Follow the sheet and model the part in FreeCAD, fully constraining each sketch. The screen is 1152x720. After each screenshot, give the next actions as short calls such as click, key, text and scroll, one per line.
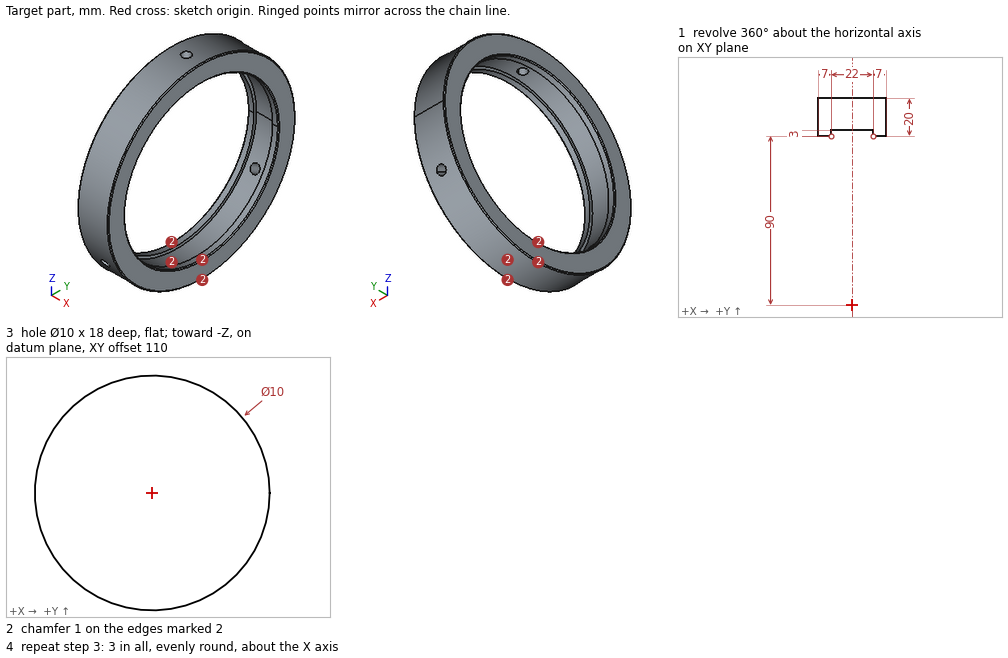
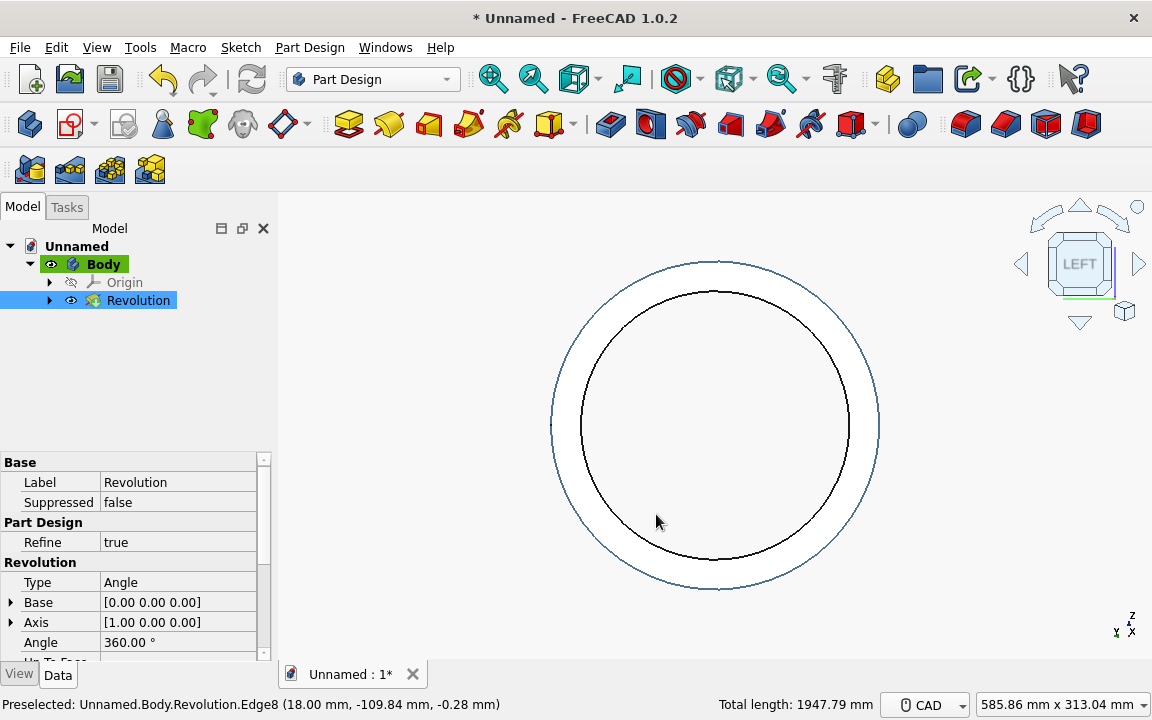
click(849, 424, ctrl)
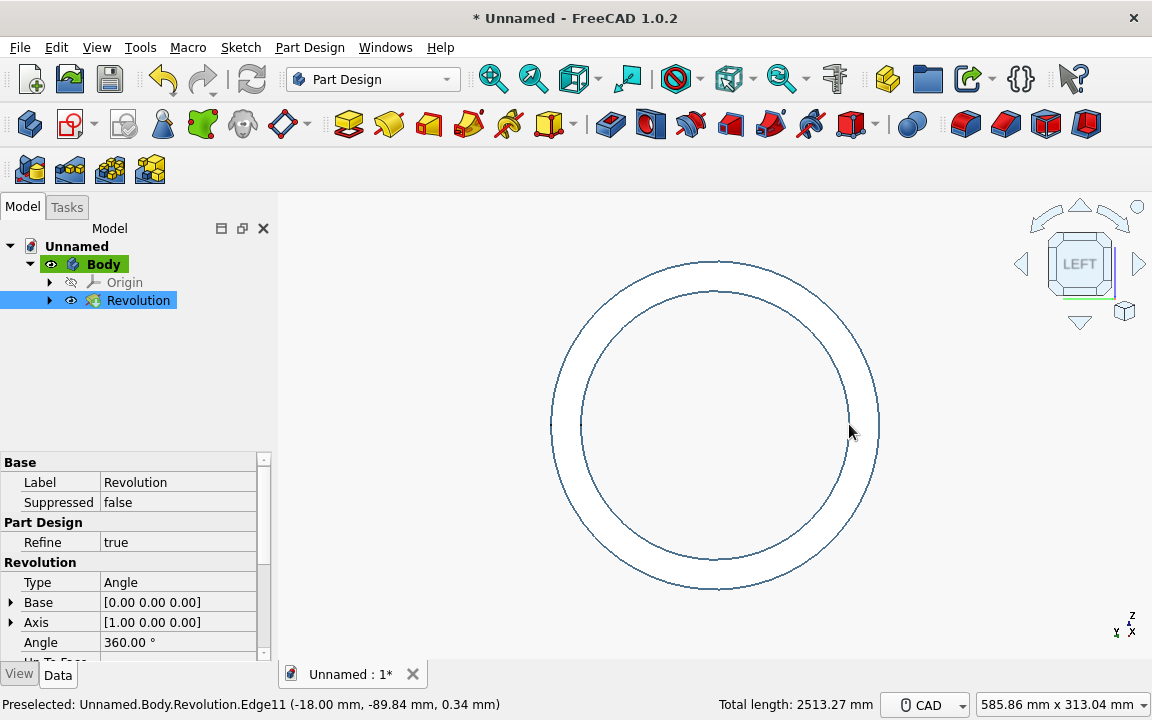
click(1006, 124)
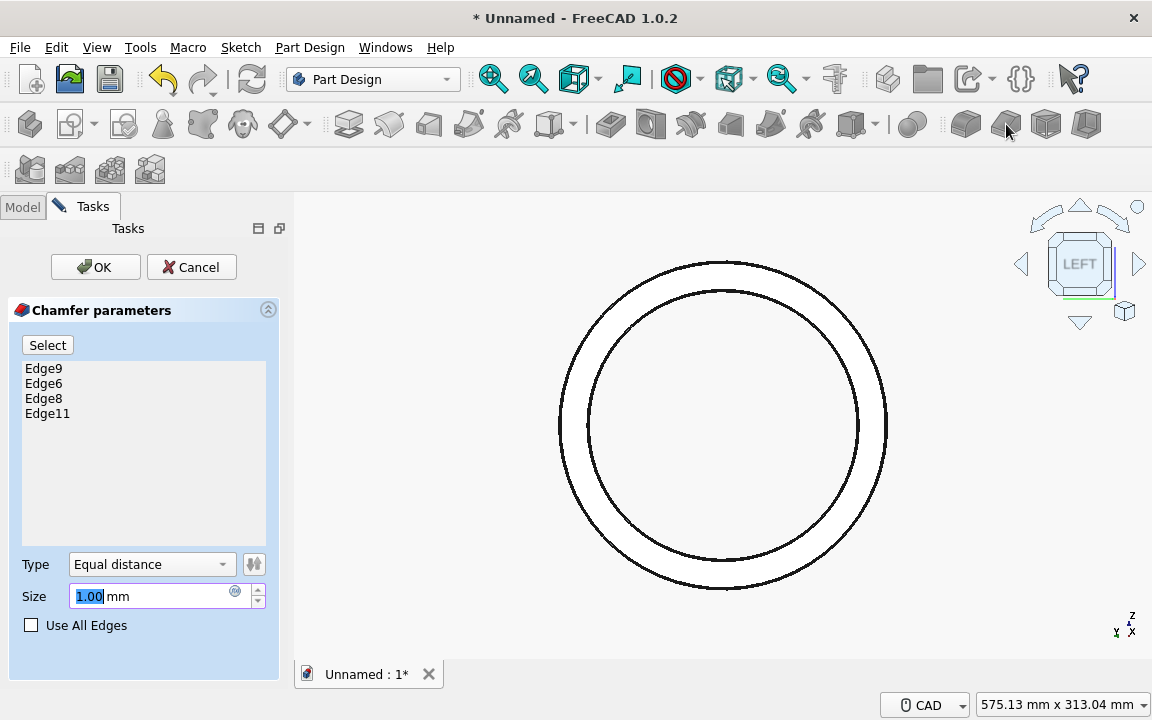
text(1)
key(Tab)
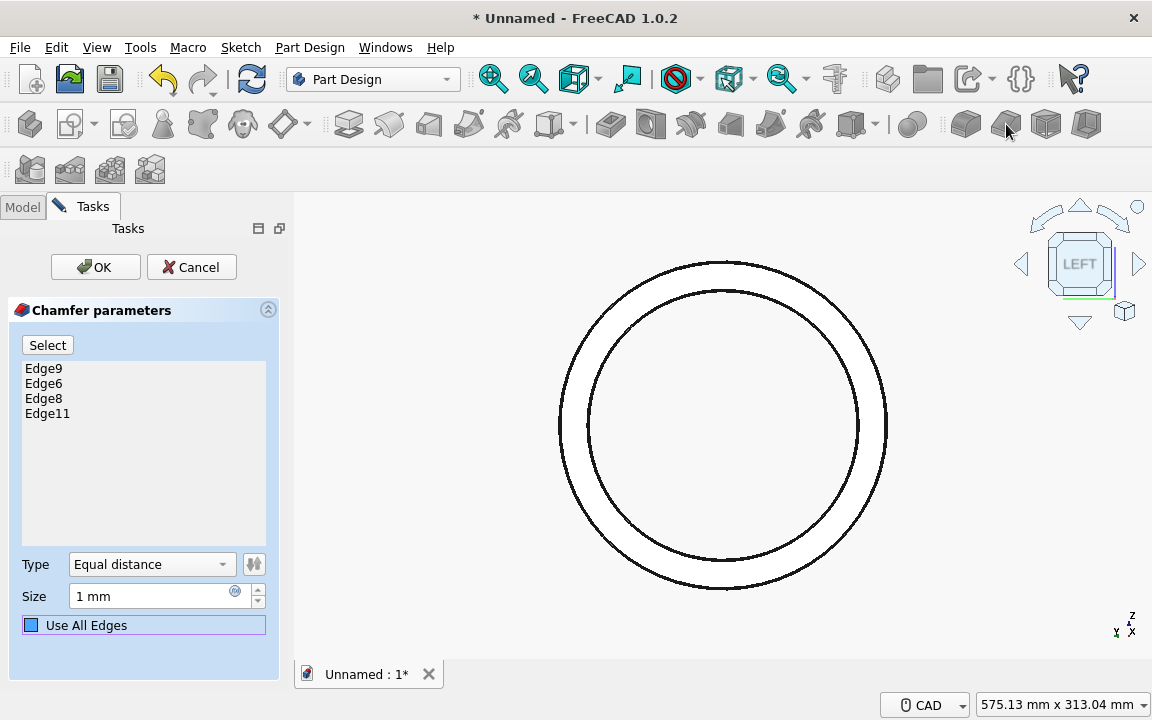
click(96, 267)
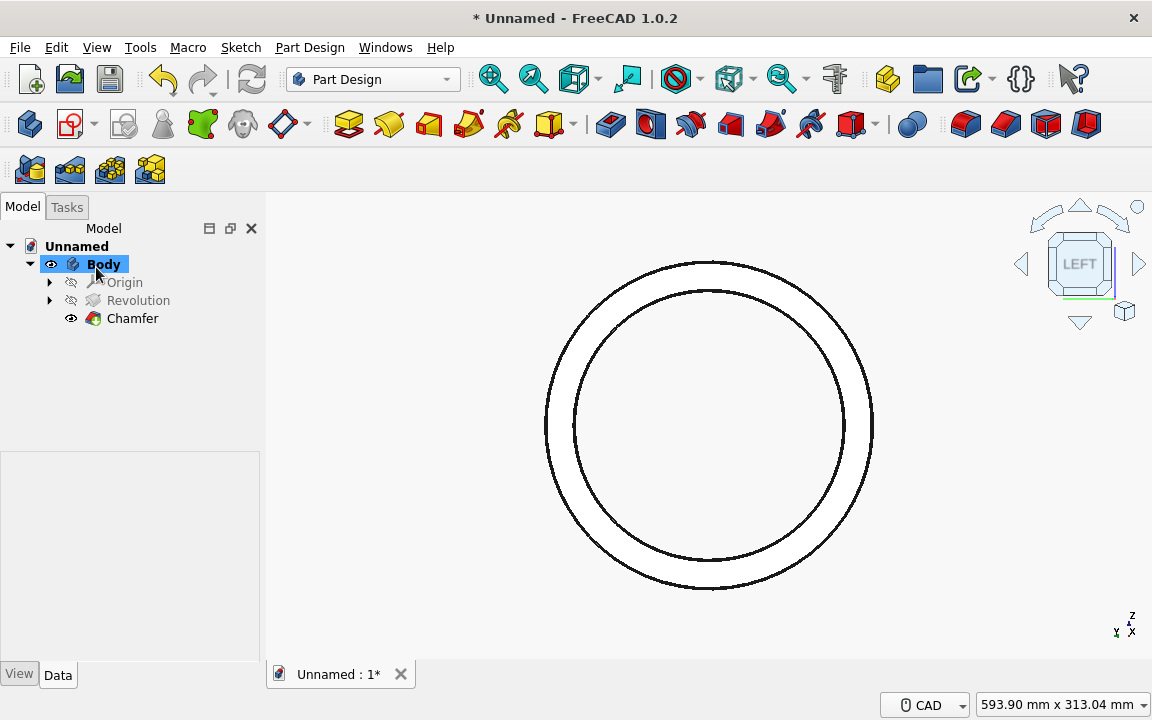
click(50, 282)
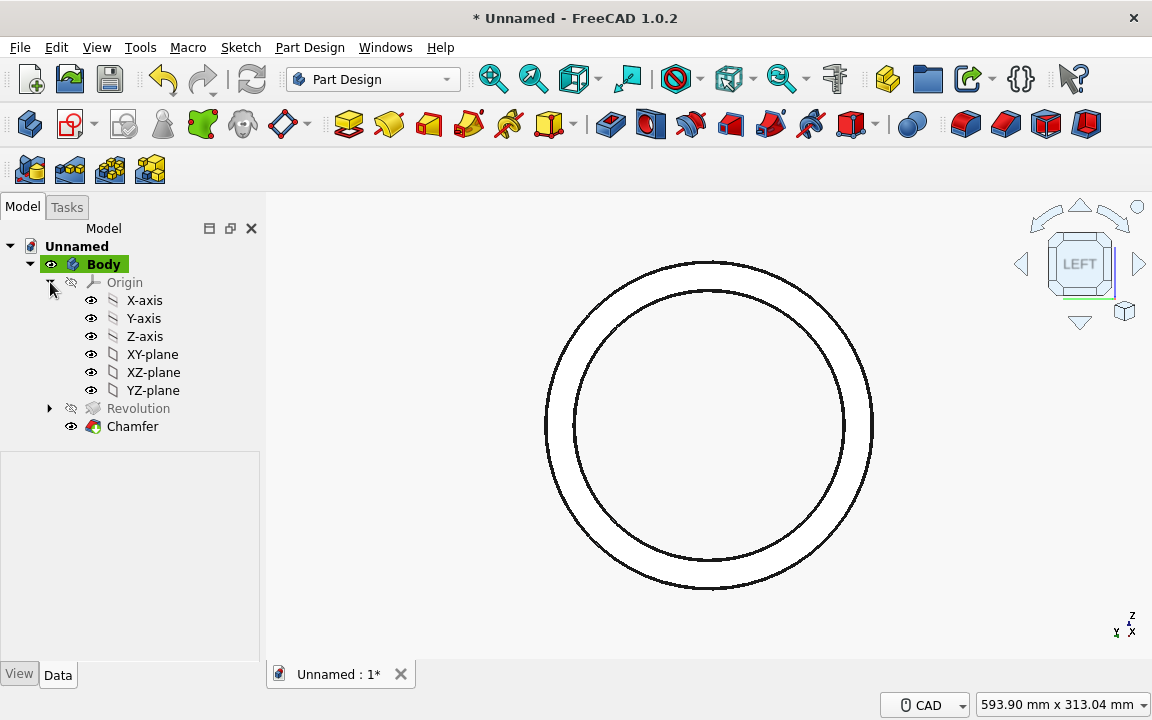
click(136, 354)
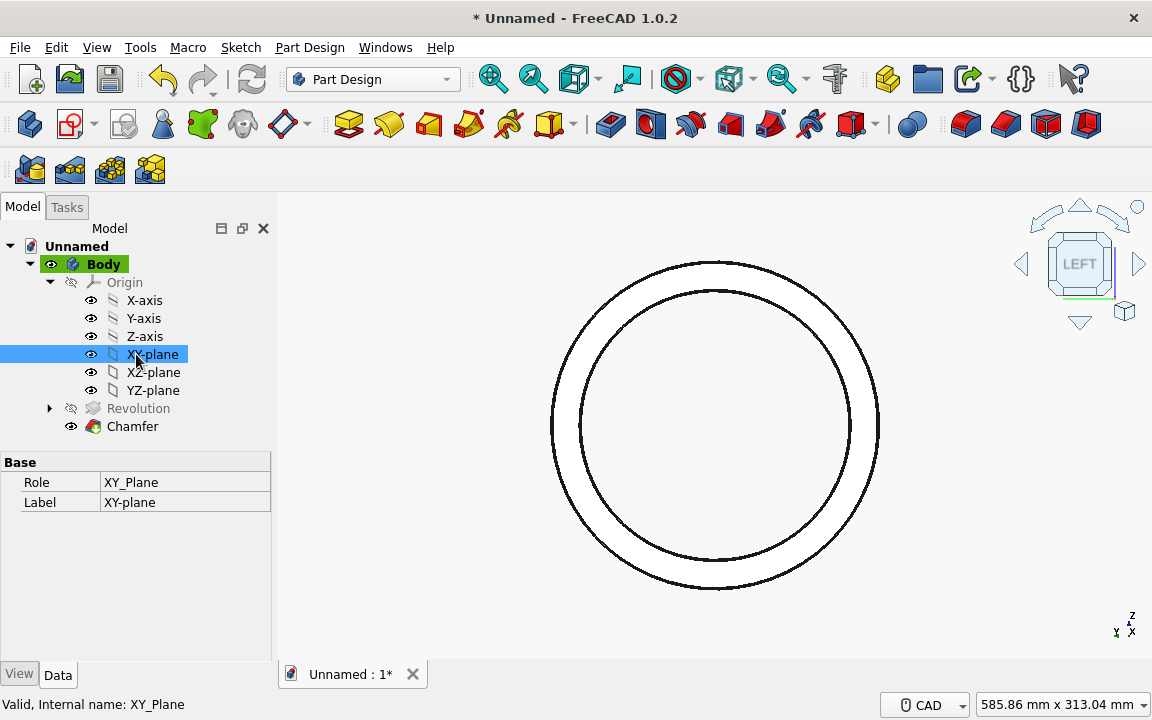
click(284, 124)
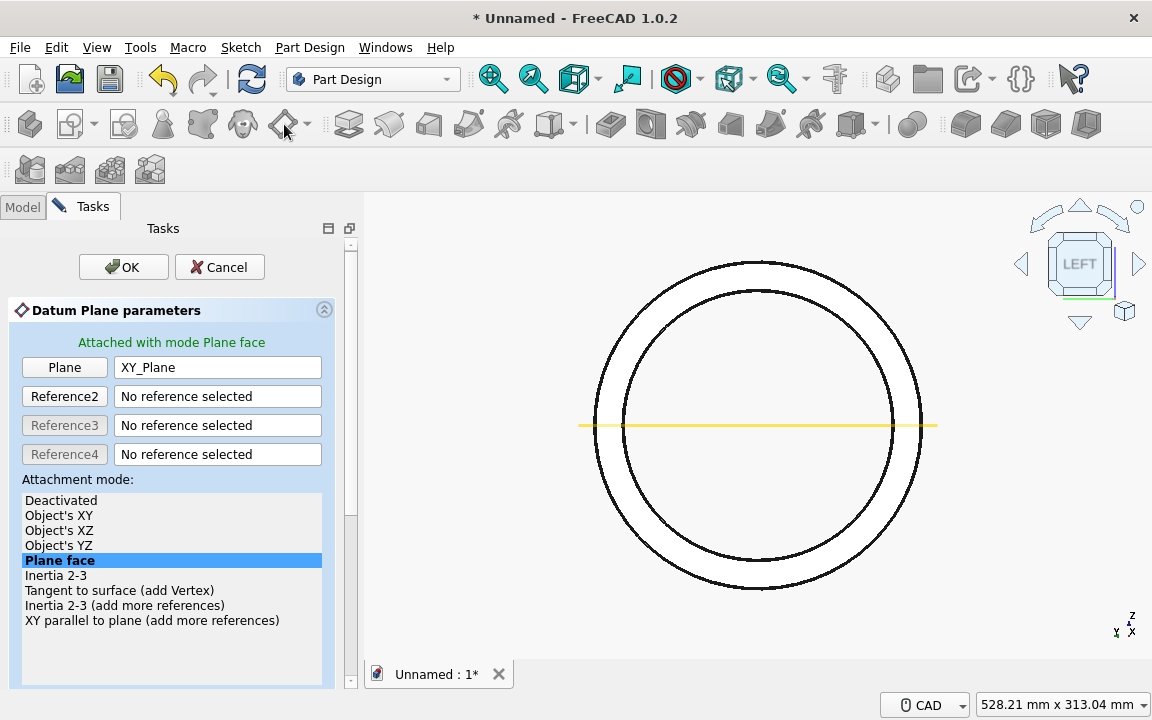
scroll(351, 463, down, 3)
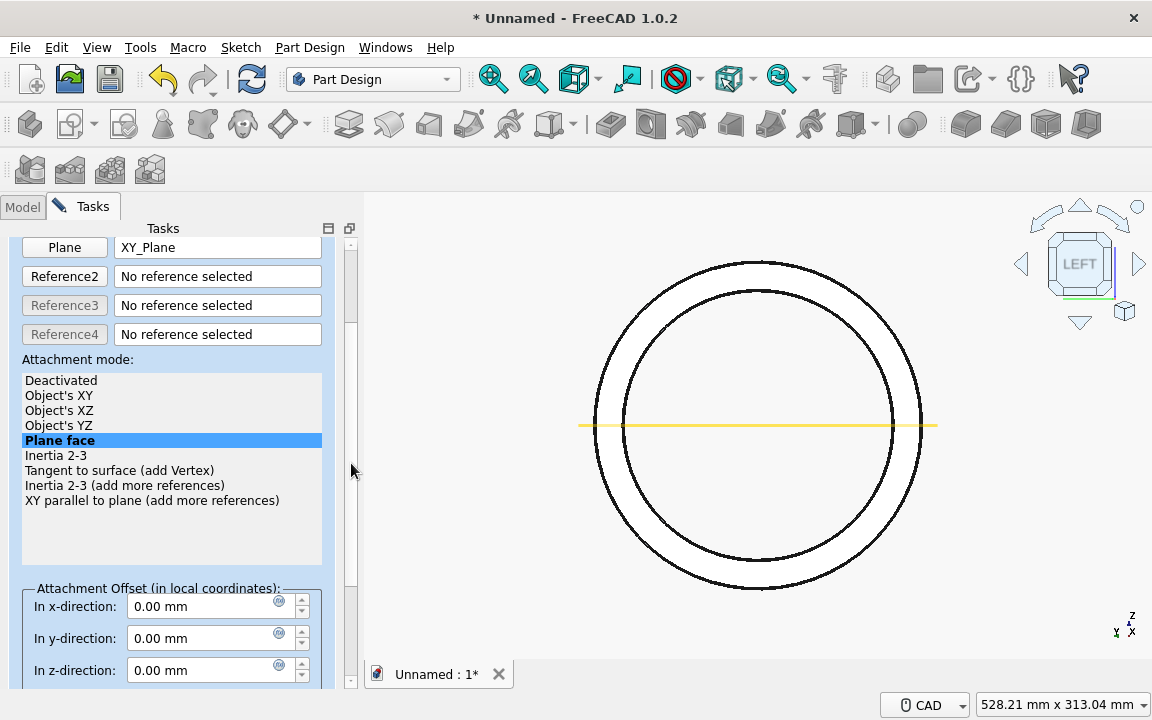
triple_click(210, 610)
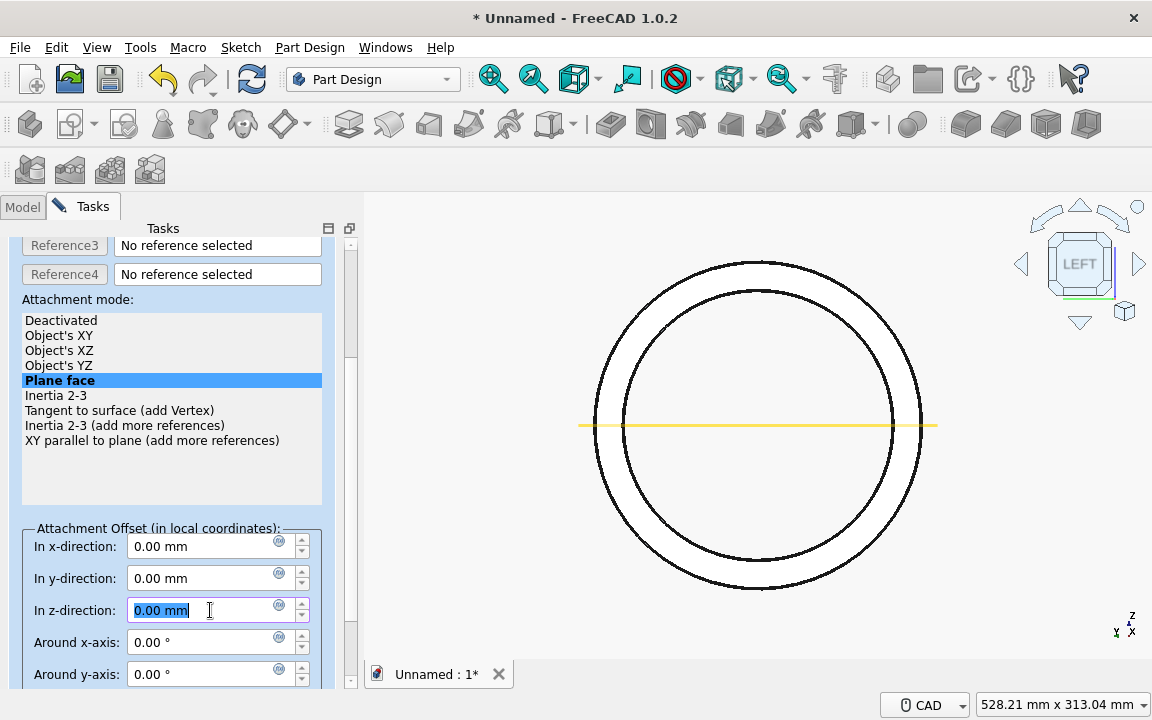
text(110)
key(Tab)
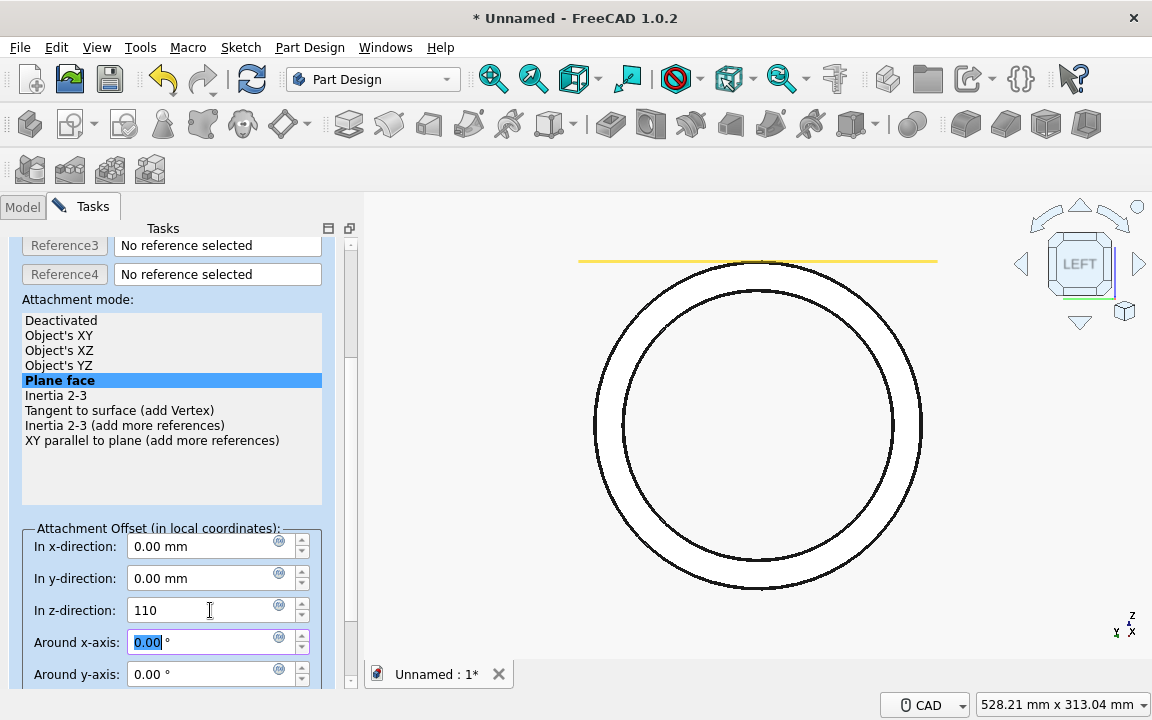
scroll(351, 463, up, 4)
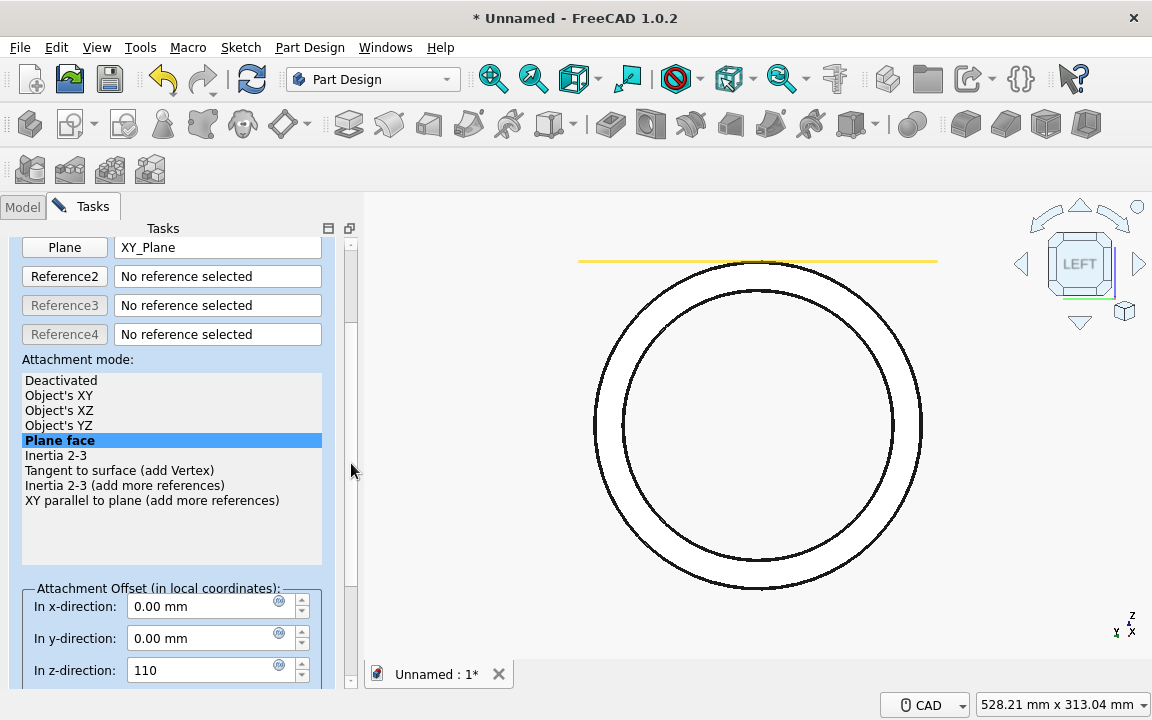
click(124, 267)